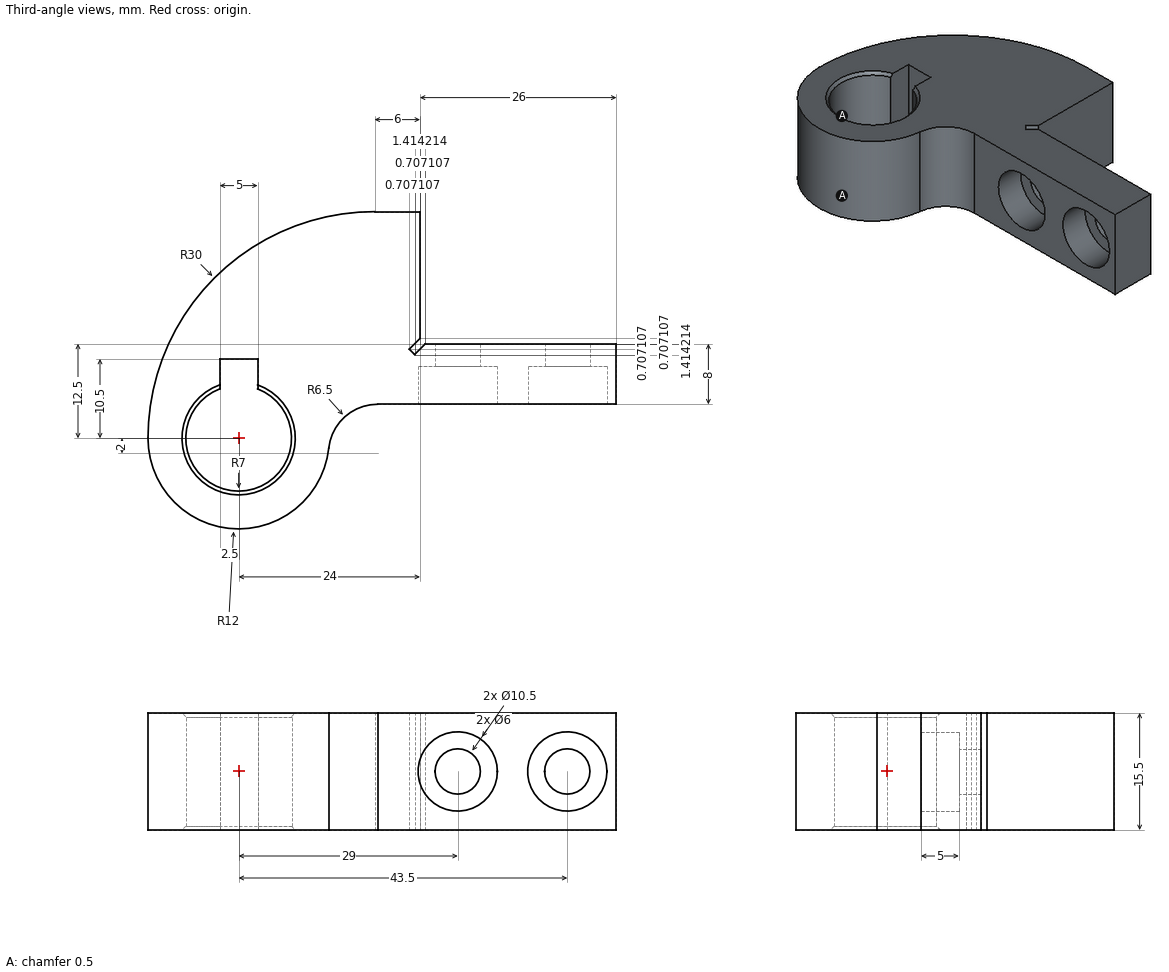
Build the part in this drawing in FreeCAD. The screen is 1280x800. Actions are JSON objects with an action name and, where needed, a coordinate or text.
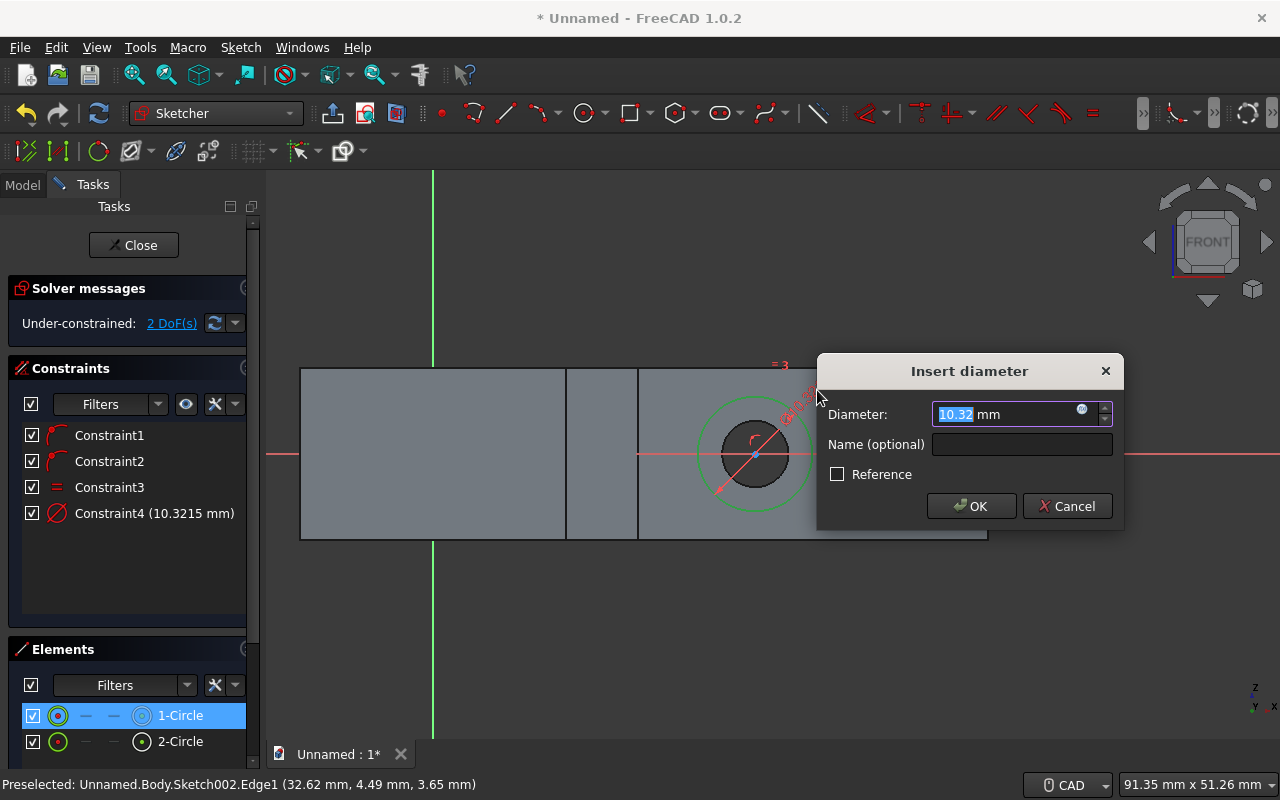
{"action": "type", "text": "10.5"}
{"action": "key", "text": "Return"}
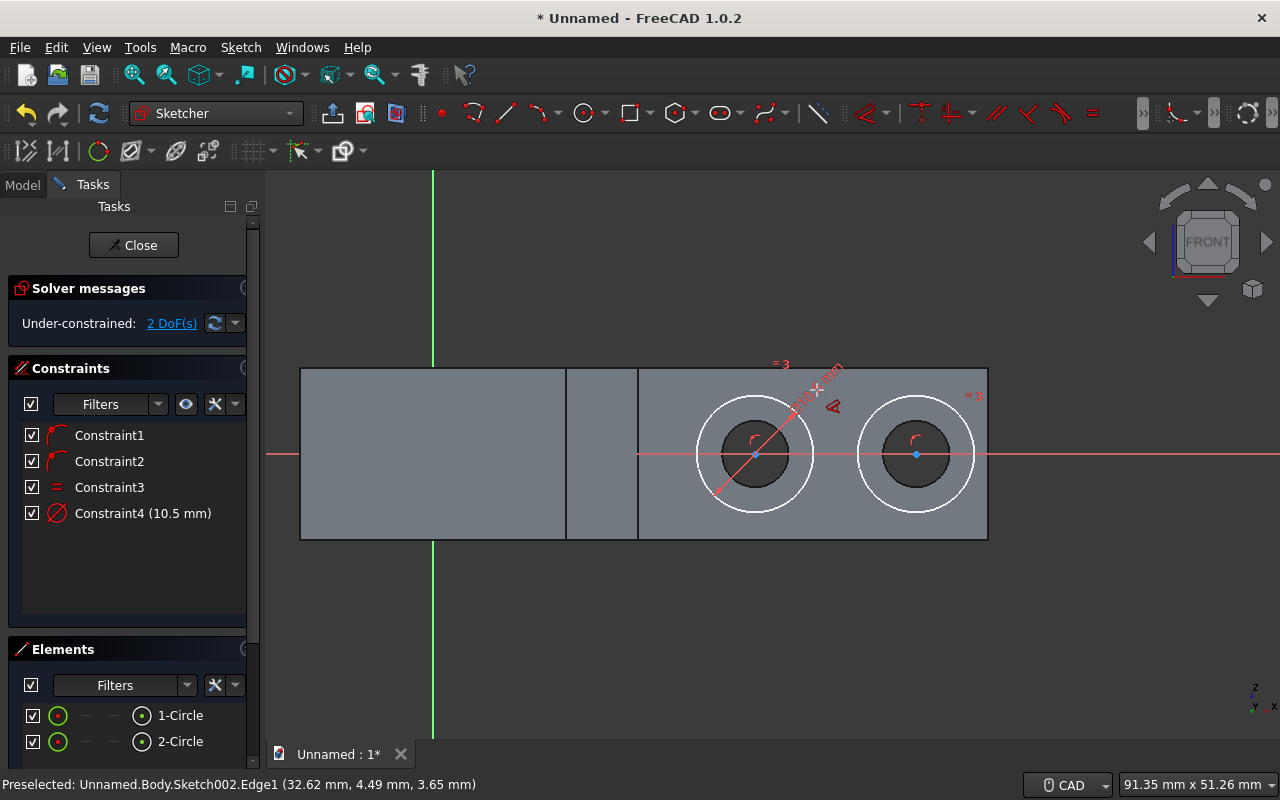
{"action": "left_click", "coordinate": [755, 454]}
{"action": "left_click", "coordinate": [594, 488]}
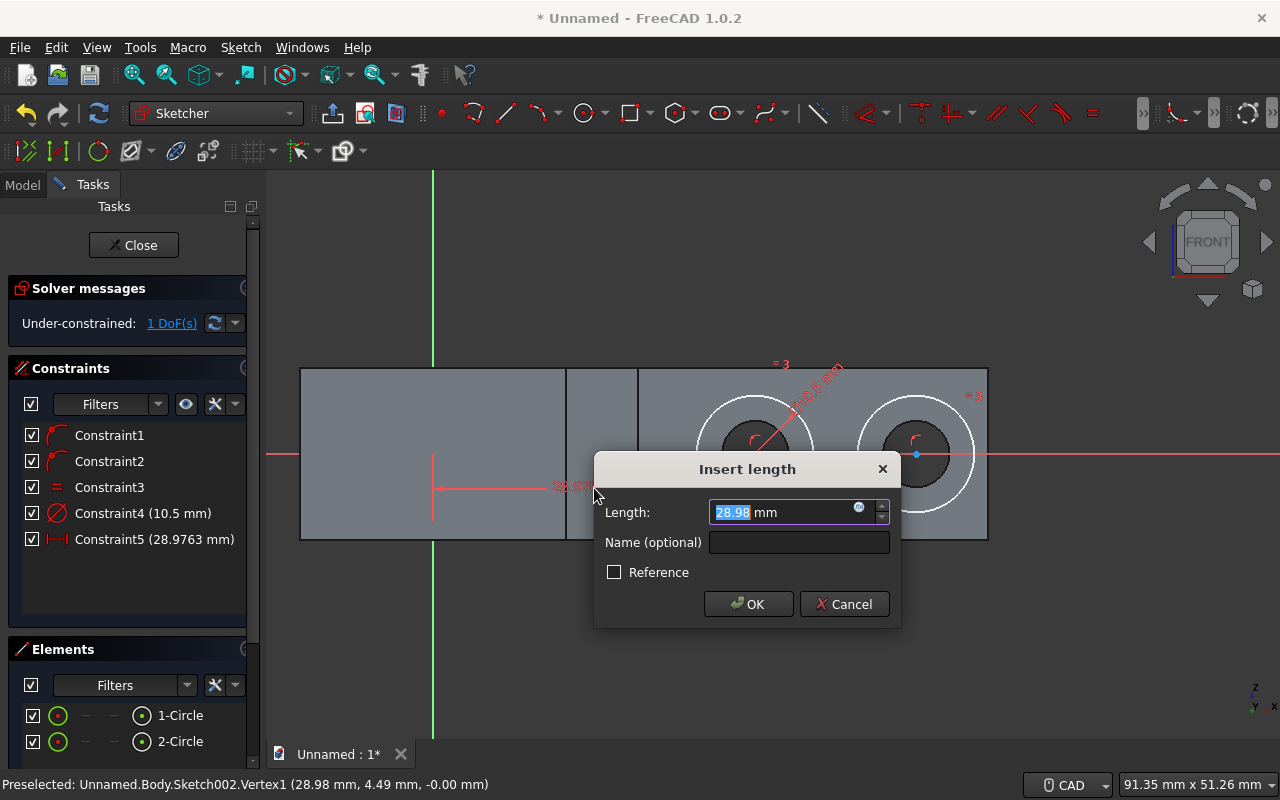
{"action": "type", "text": "29"}
{"action": "key", "text": "Return"}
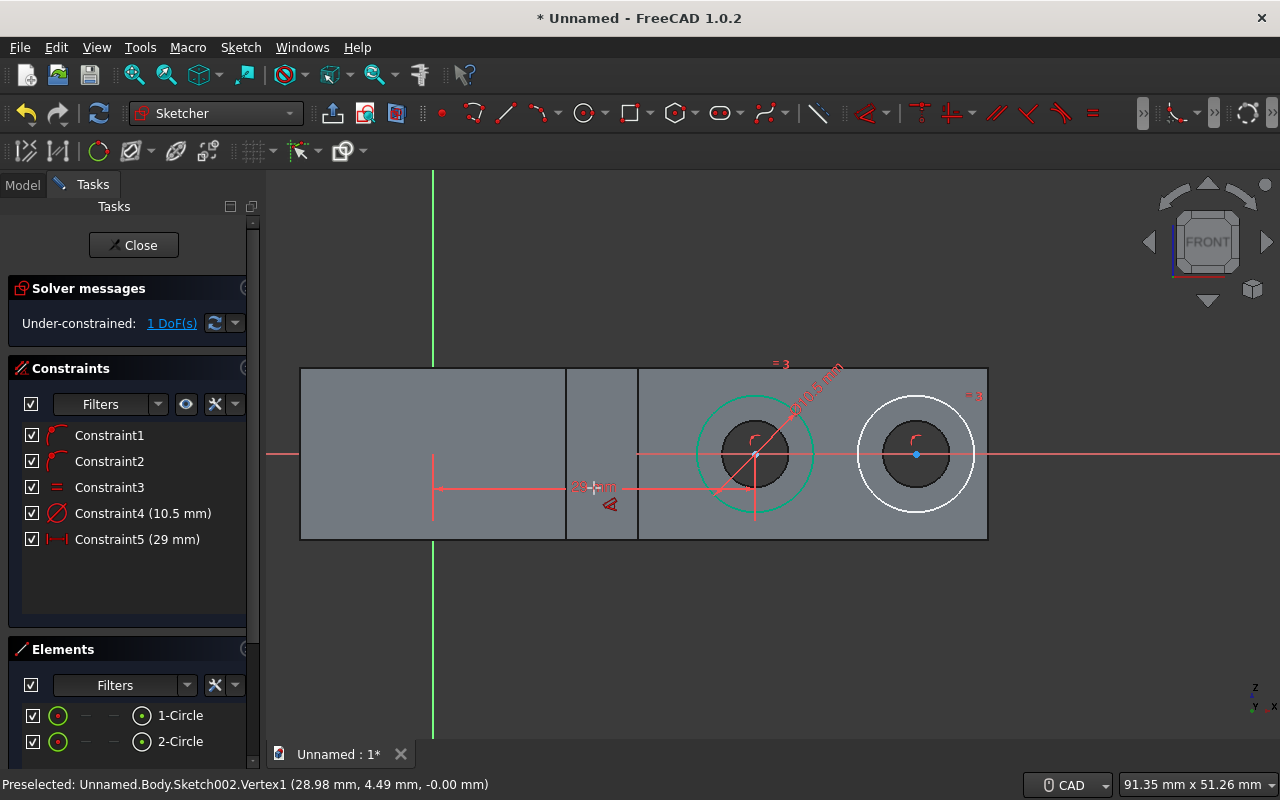
{"action": "left_click", "coordinate": [916, 454]}
{"action": "left_click", "coordinate": [675, 488]}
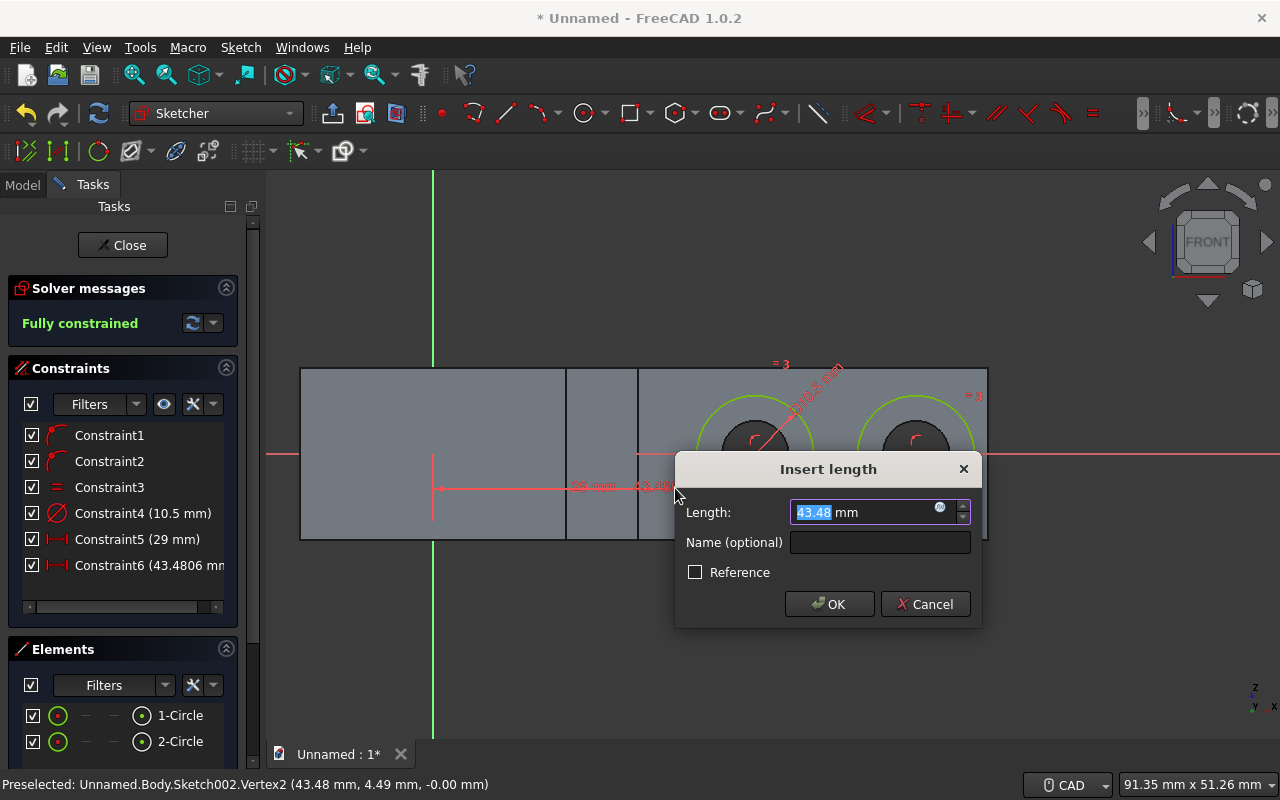
{"action": "type", "text": "43.5"}
{"action": "key", "text": "Return"}
{"action": "key", "text": "Escape"}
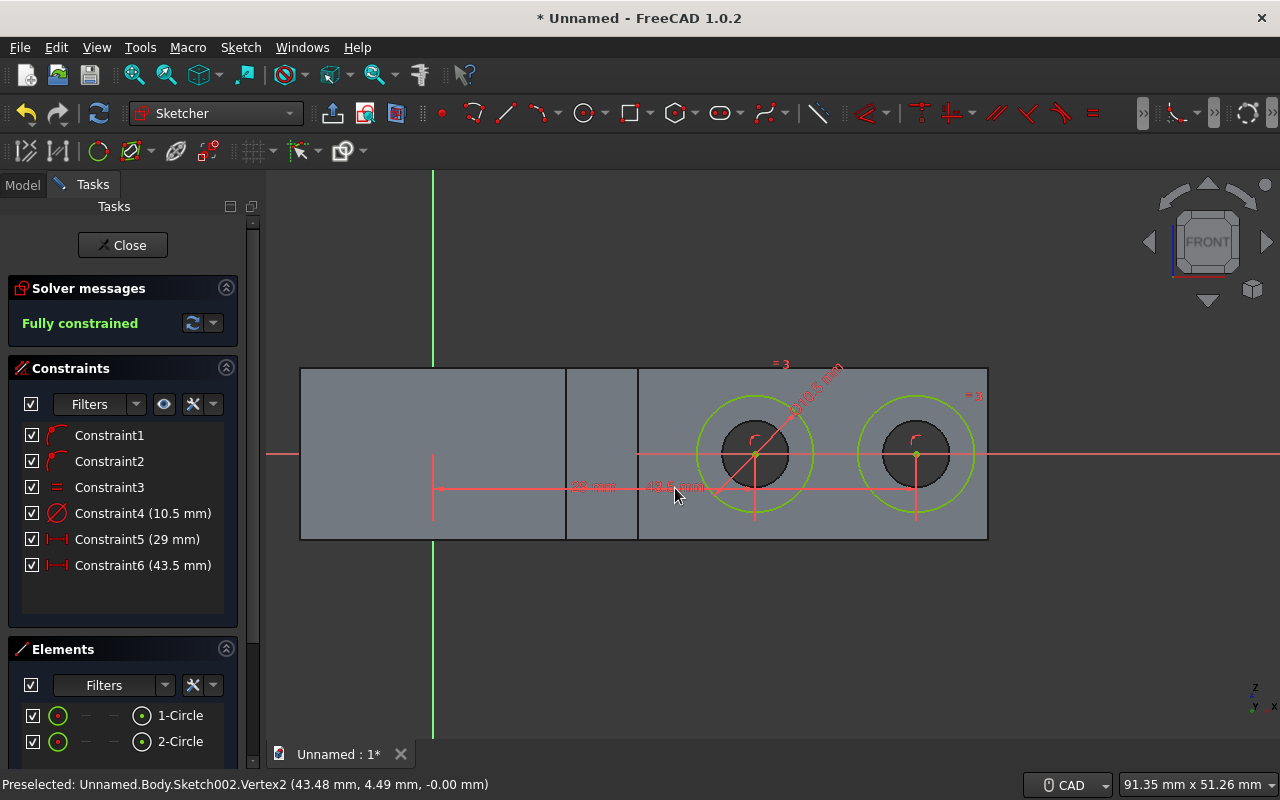
{"action": "left_click", "coordinate": [123, 245]}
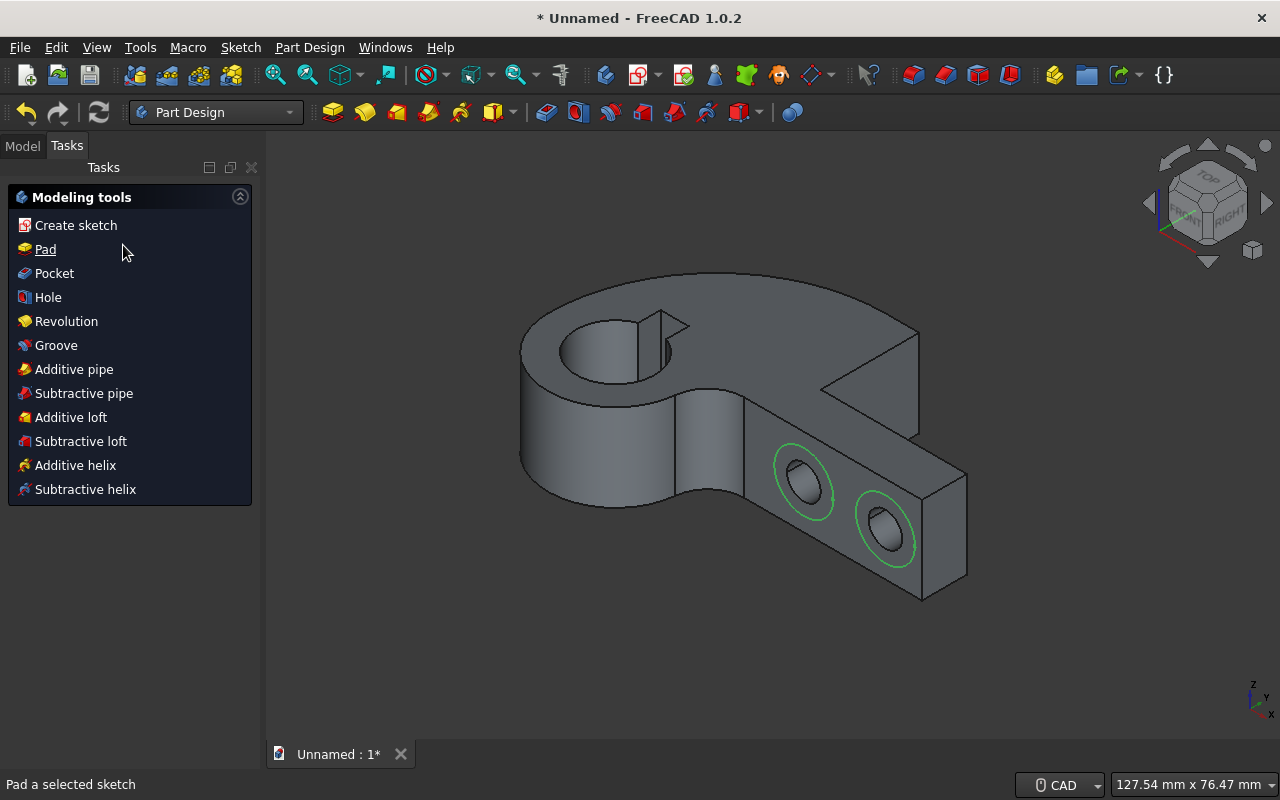
{"action": "left_click", "coordinate": [548, 112]}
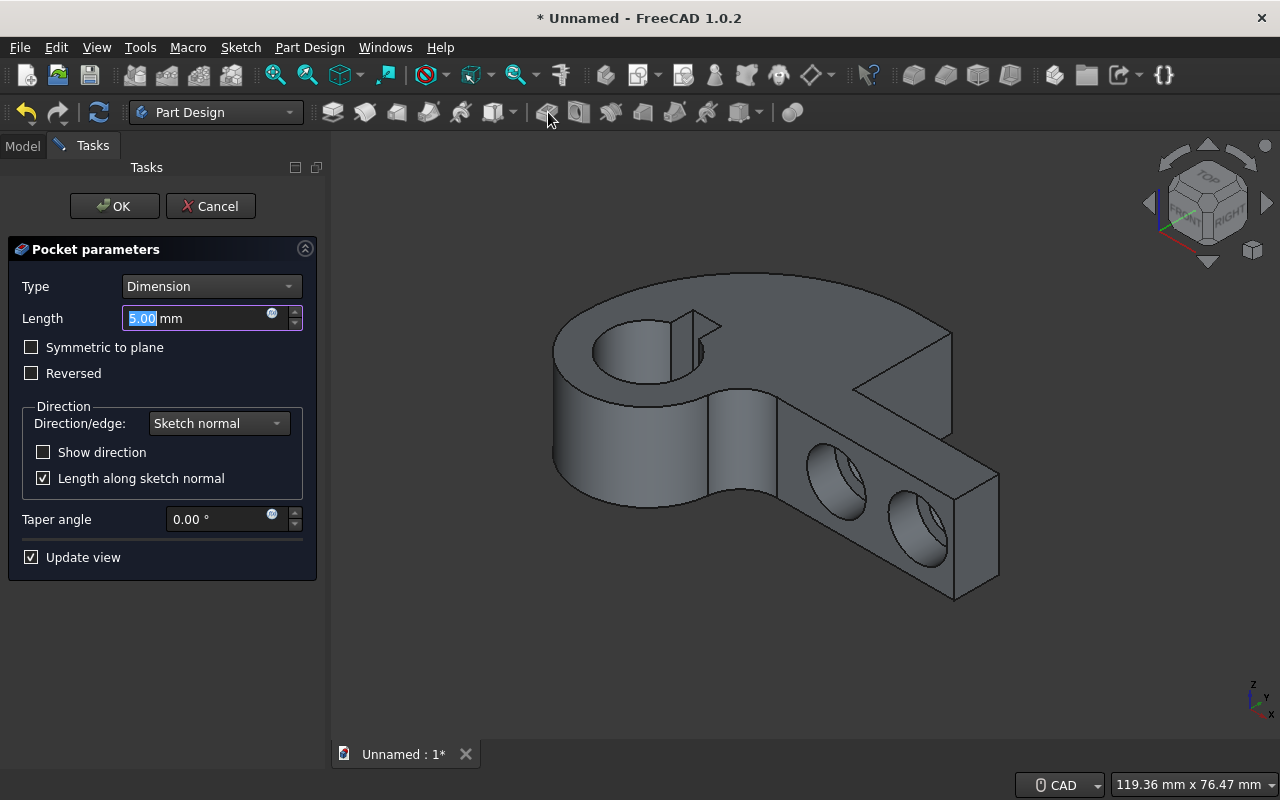
{"action": "type", "text": "5"}
{"action": "key", "text": "Tab"}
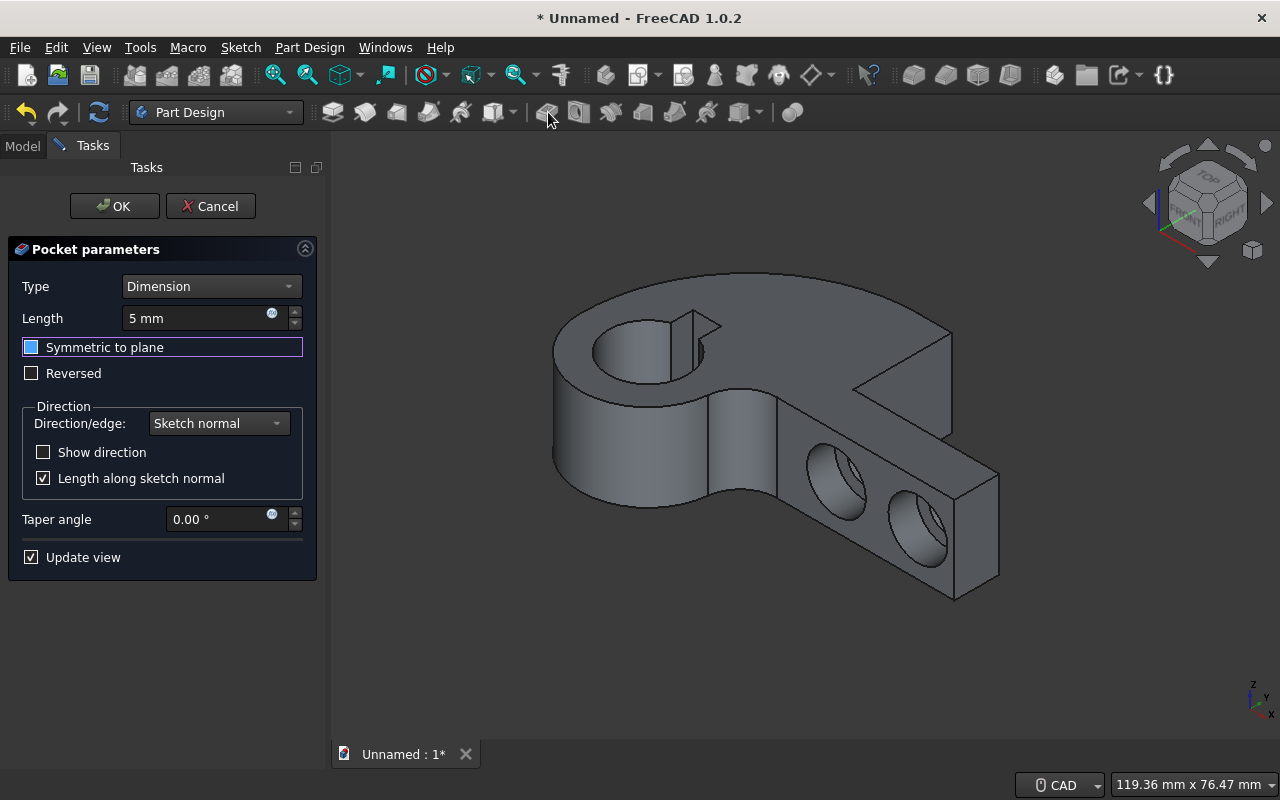
{"action": "left_click", "coordinate": [115, 206]}